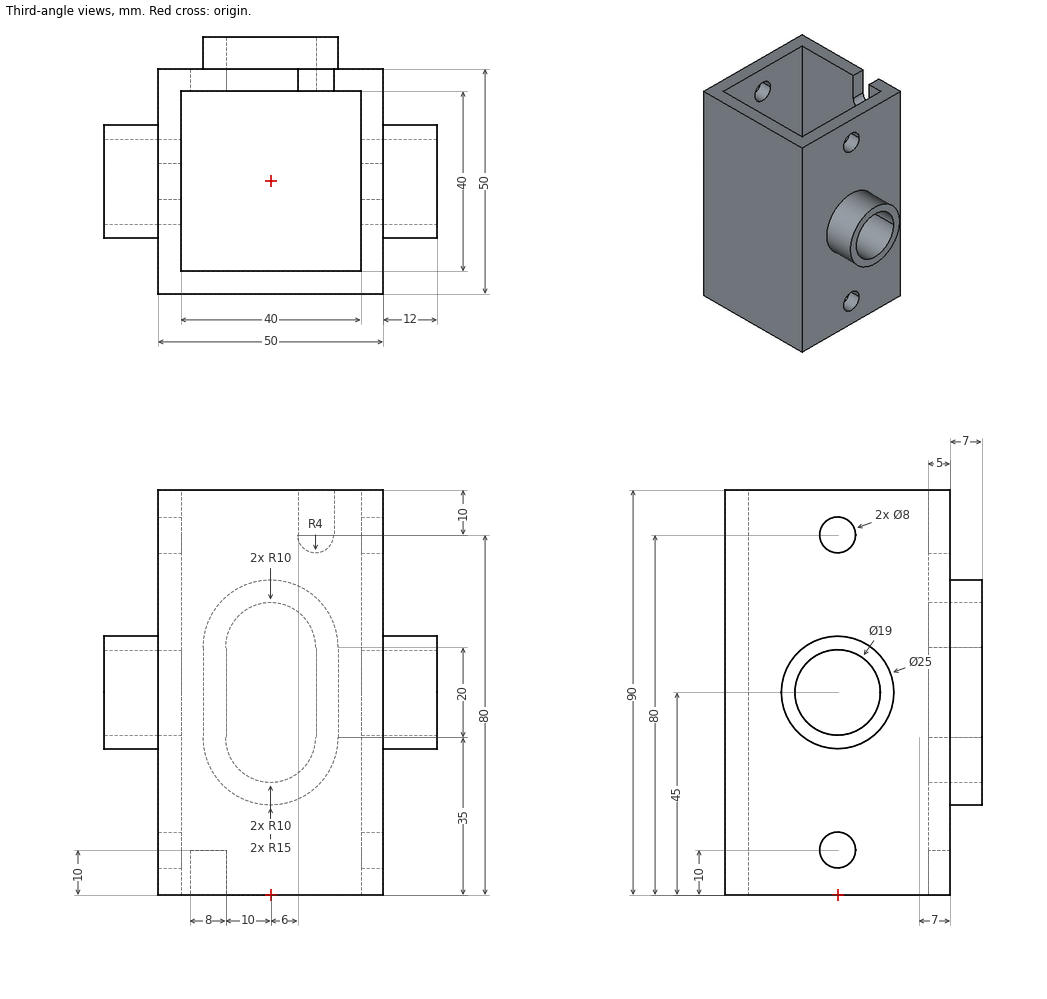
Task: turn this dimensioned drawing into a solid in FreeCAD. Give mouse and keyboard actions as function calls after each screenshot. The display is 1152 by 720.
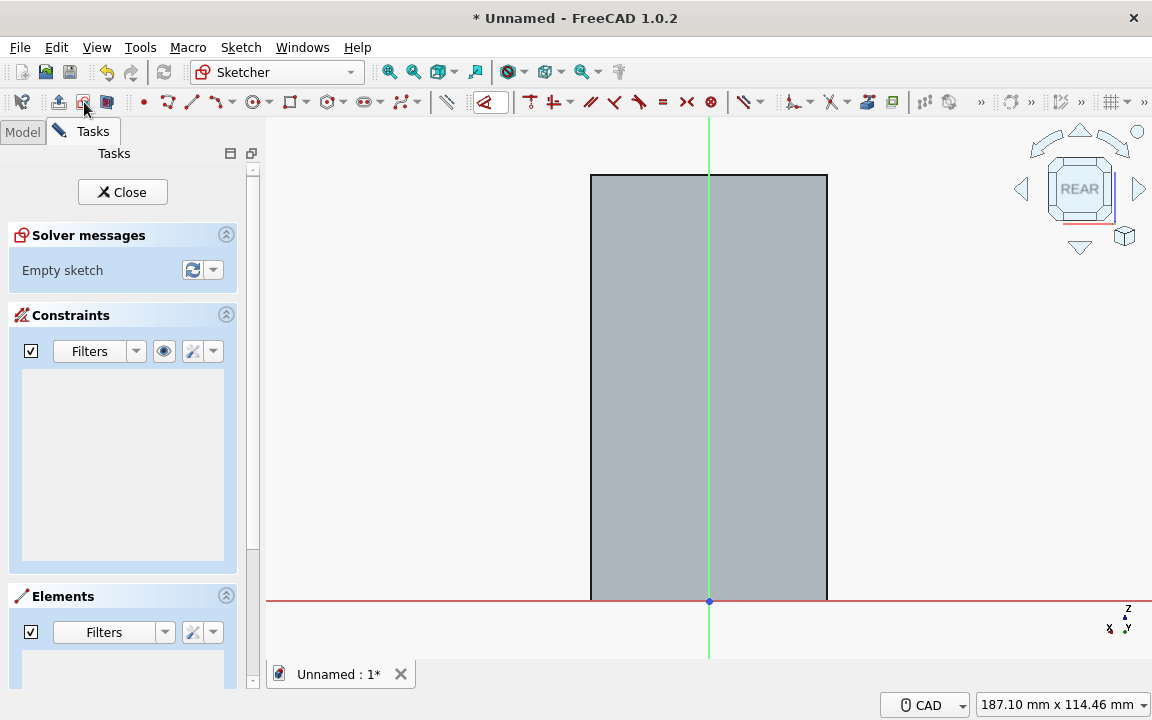
click(168, 102)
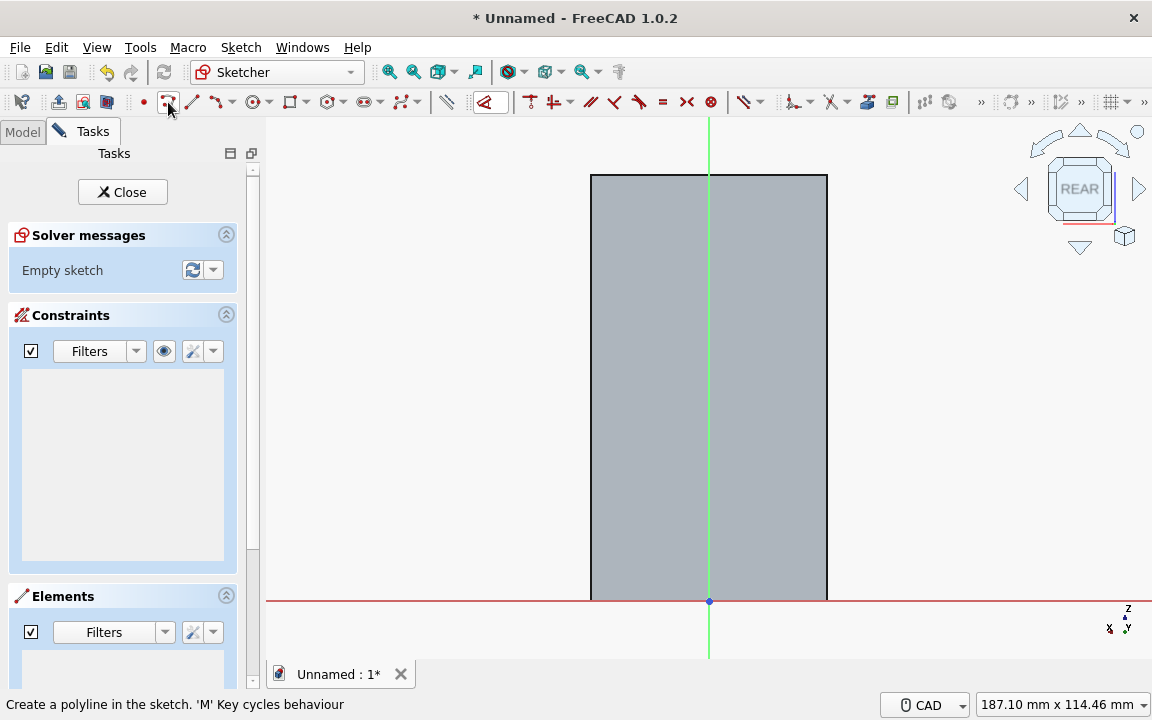
click(681, 222)
click(681, 175)
click(643, 175)
click(643, 222)
right_click(643, 222)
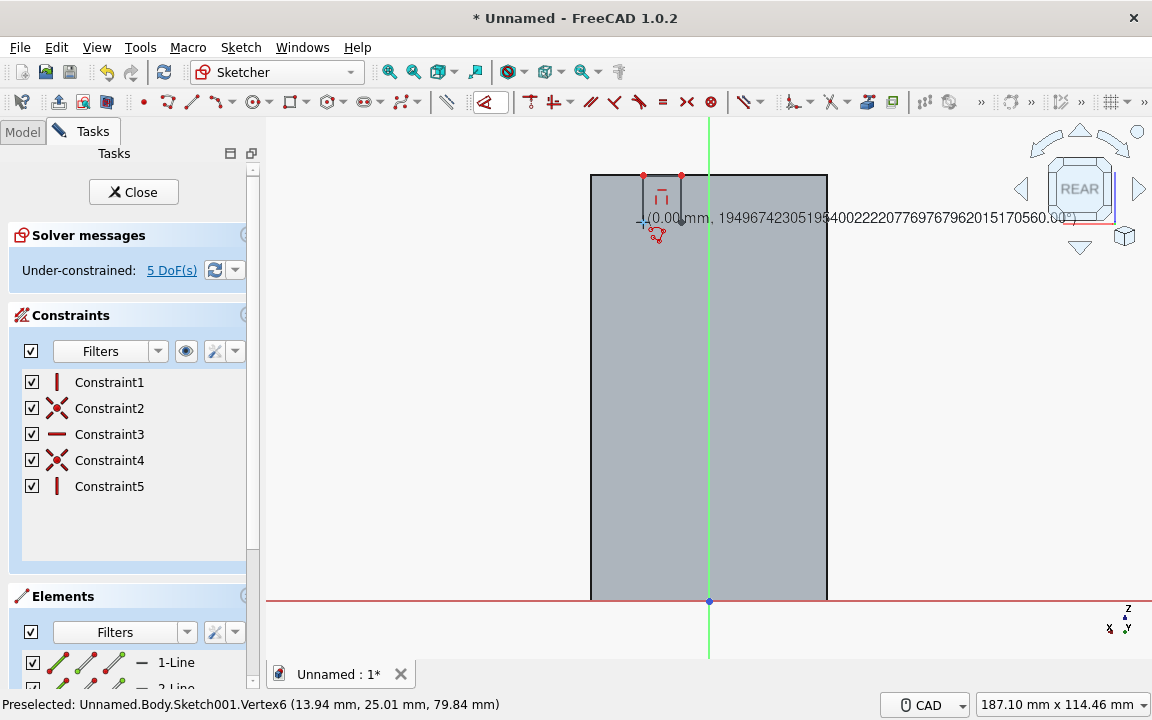
key(g)
key(3)
key(a)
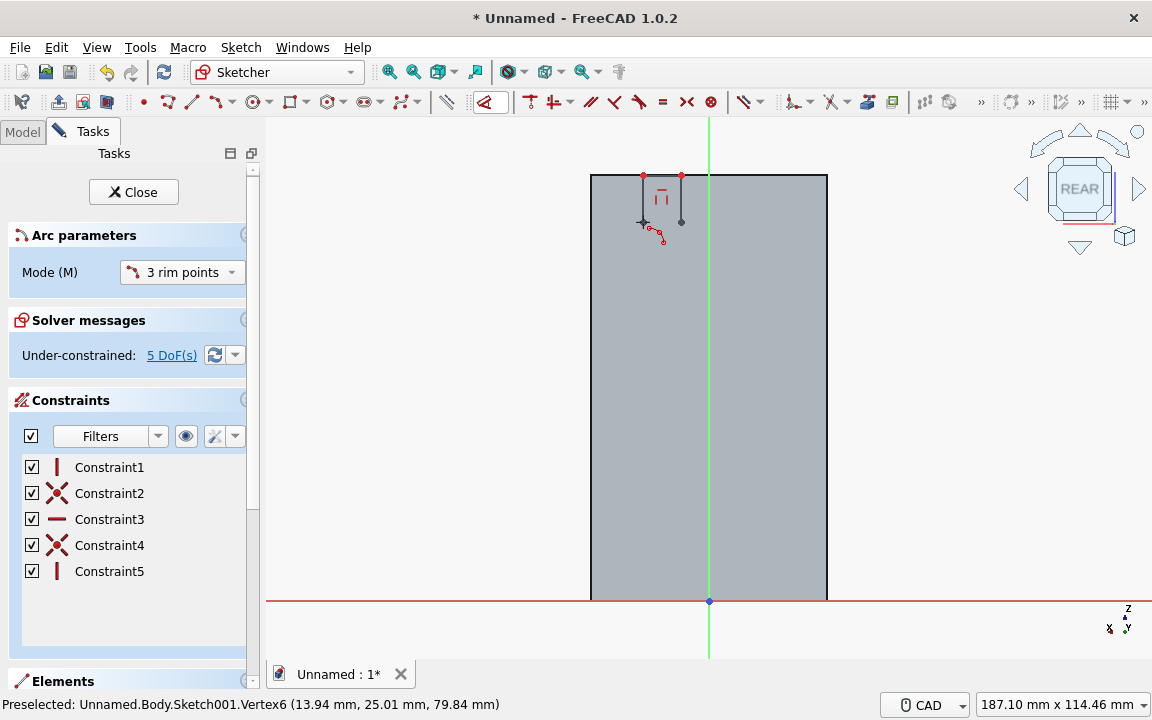
click(643, 223)
click(681, 223)
click(662, 241)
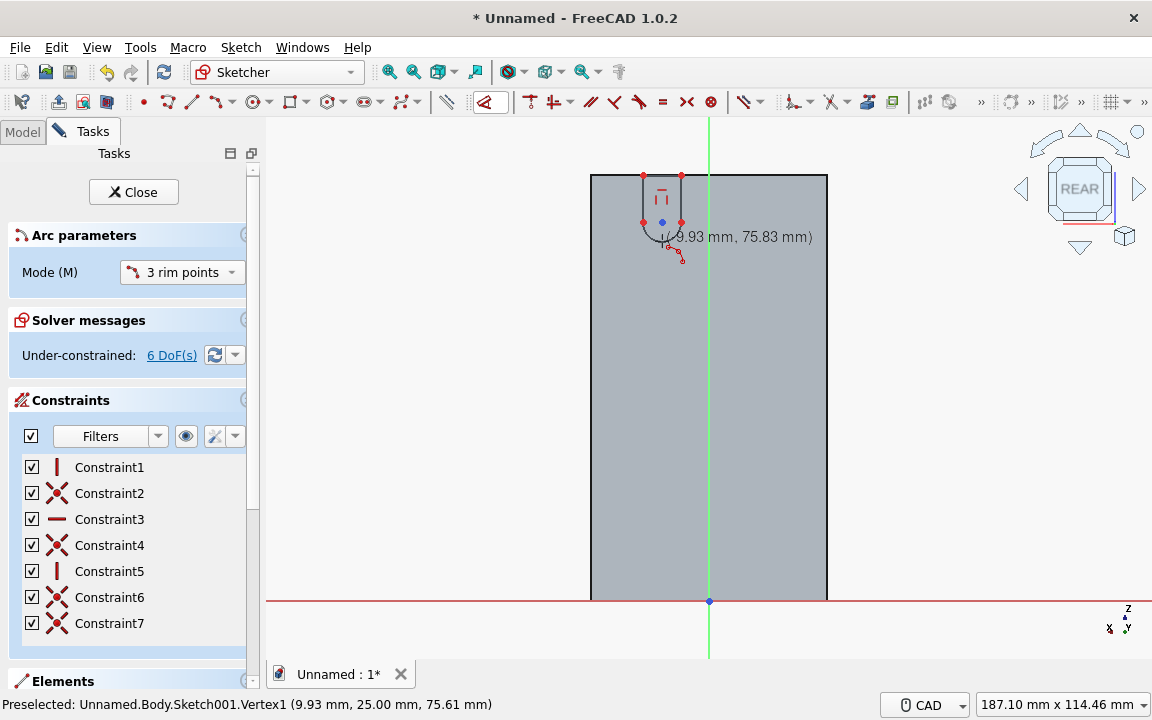
key(g)
key(r)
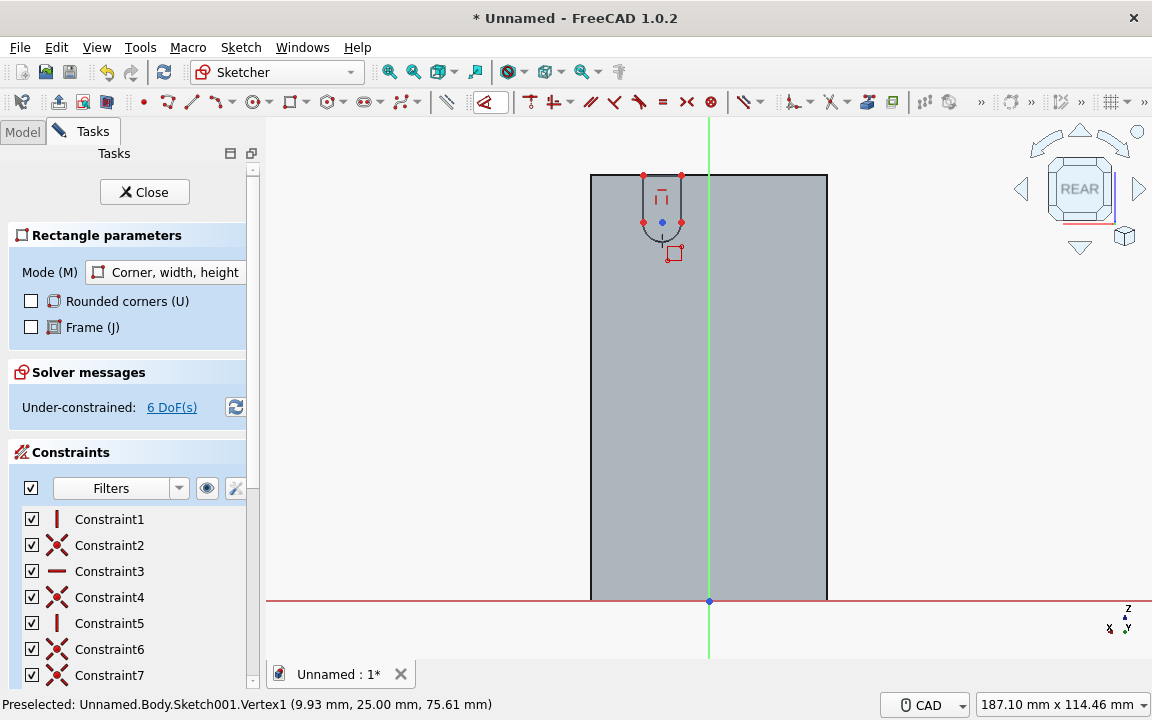
click(756, 554)
click(794, 601)
key(Escape)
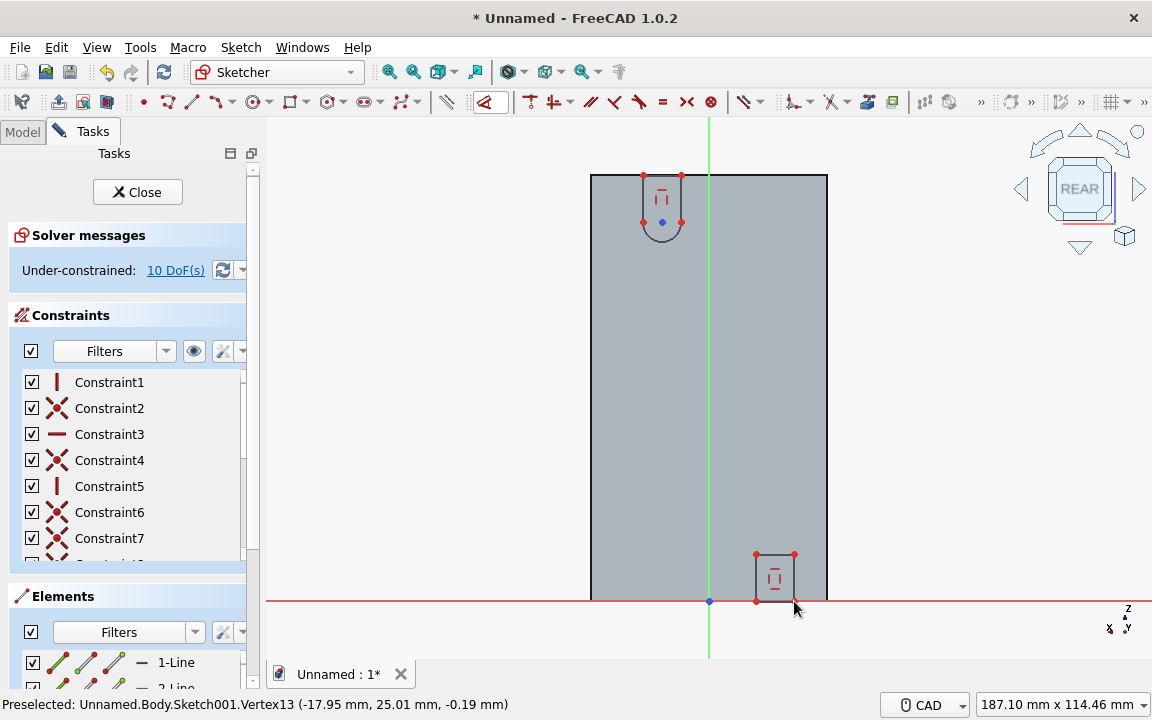
click(681, 209)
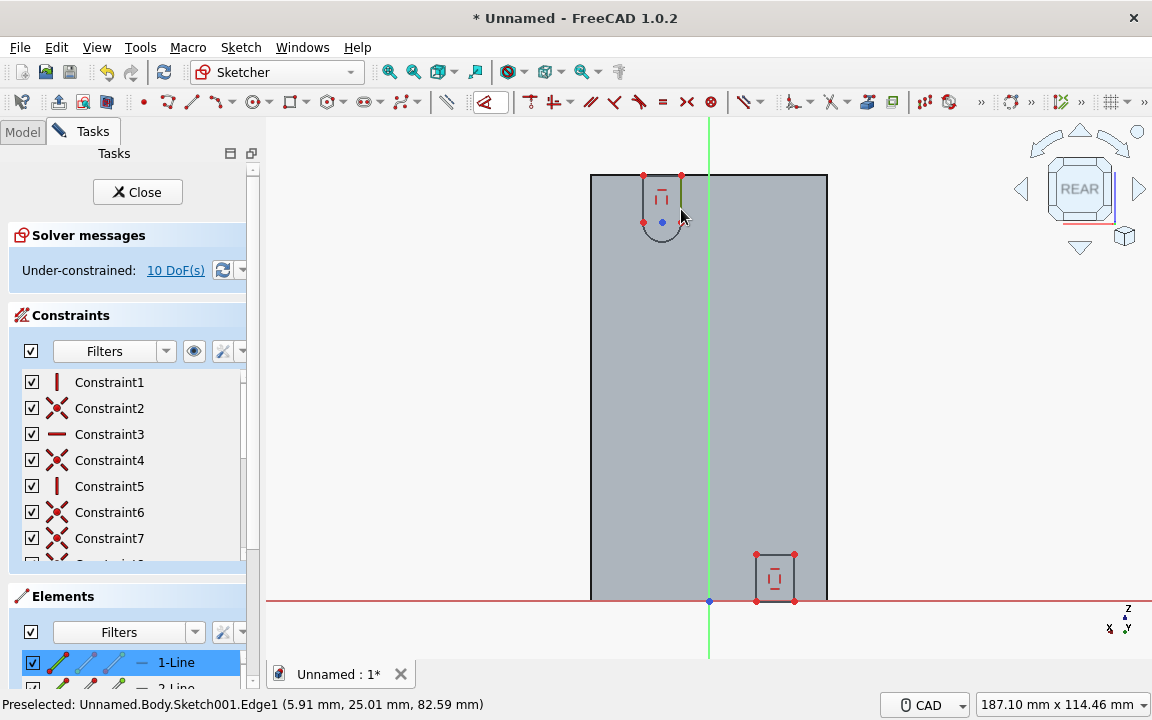
click(651, 238)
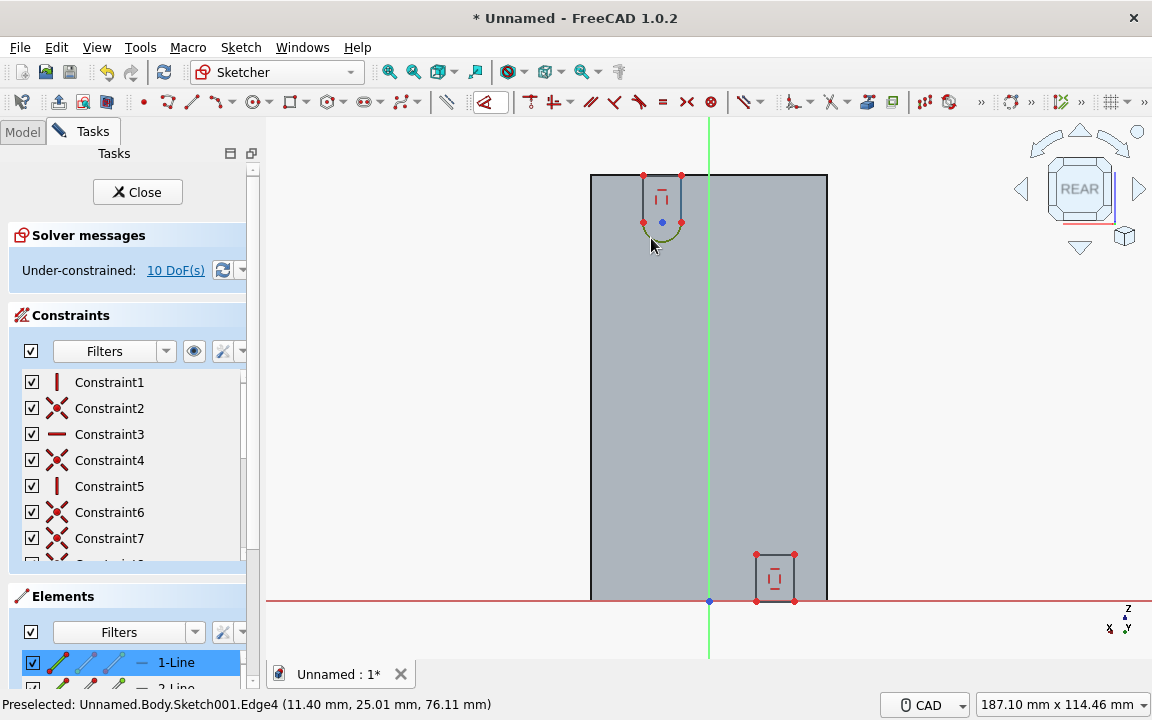
key(t)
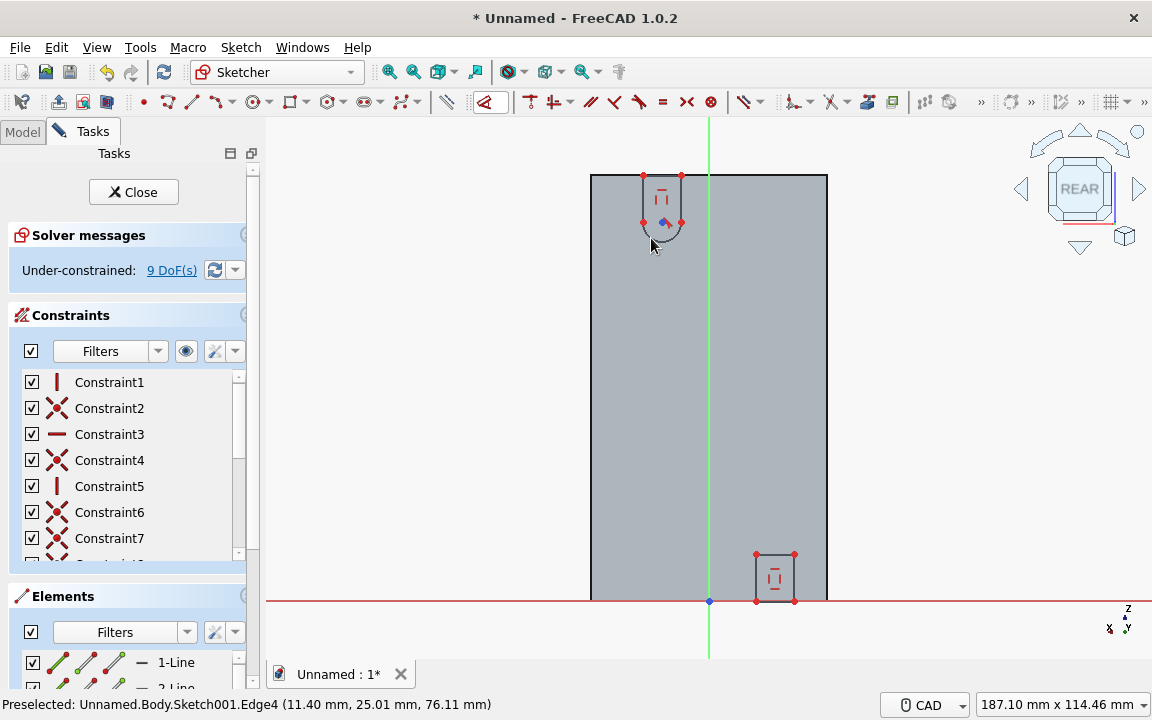
click(643, 190)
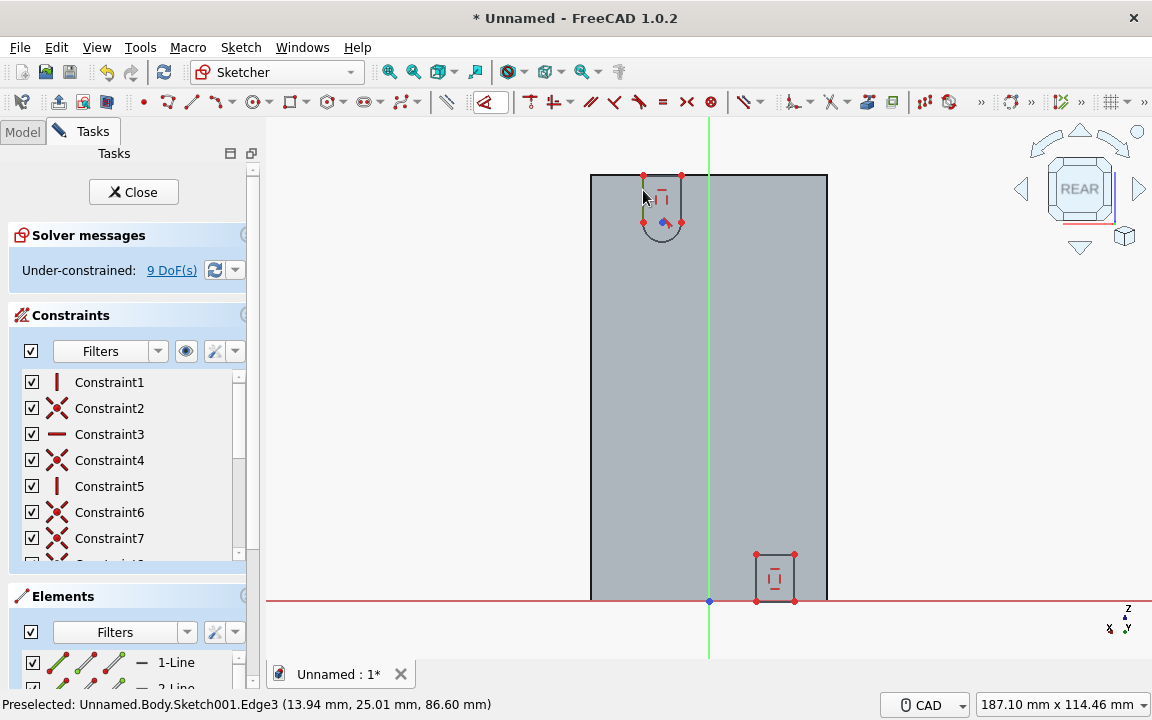
click(651, 238)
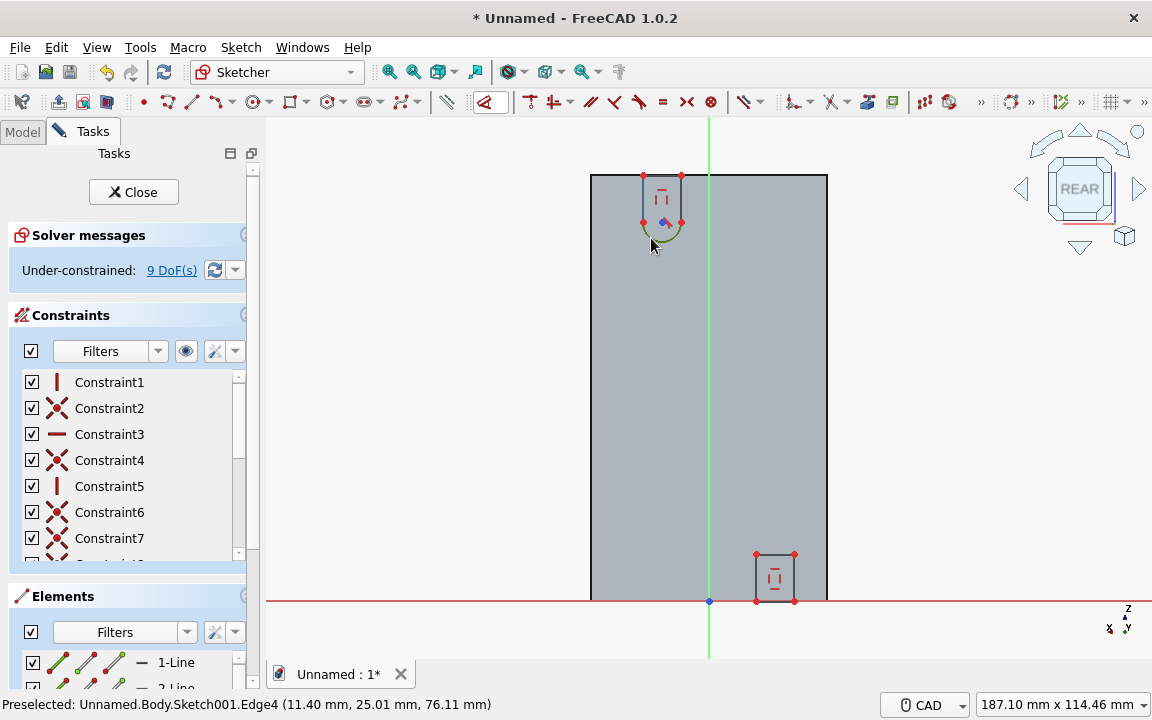
click(640, 102)